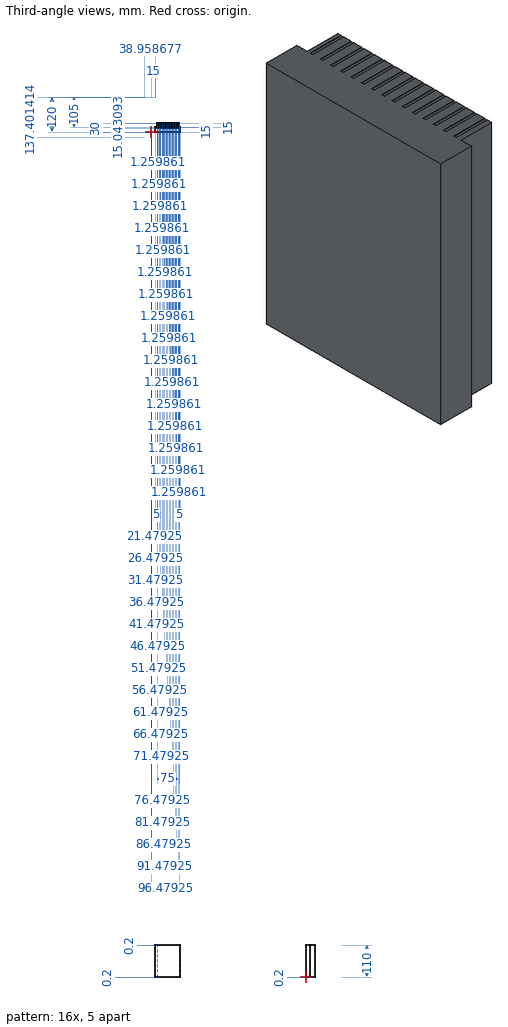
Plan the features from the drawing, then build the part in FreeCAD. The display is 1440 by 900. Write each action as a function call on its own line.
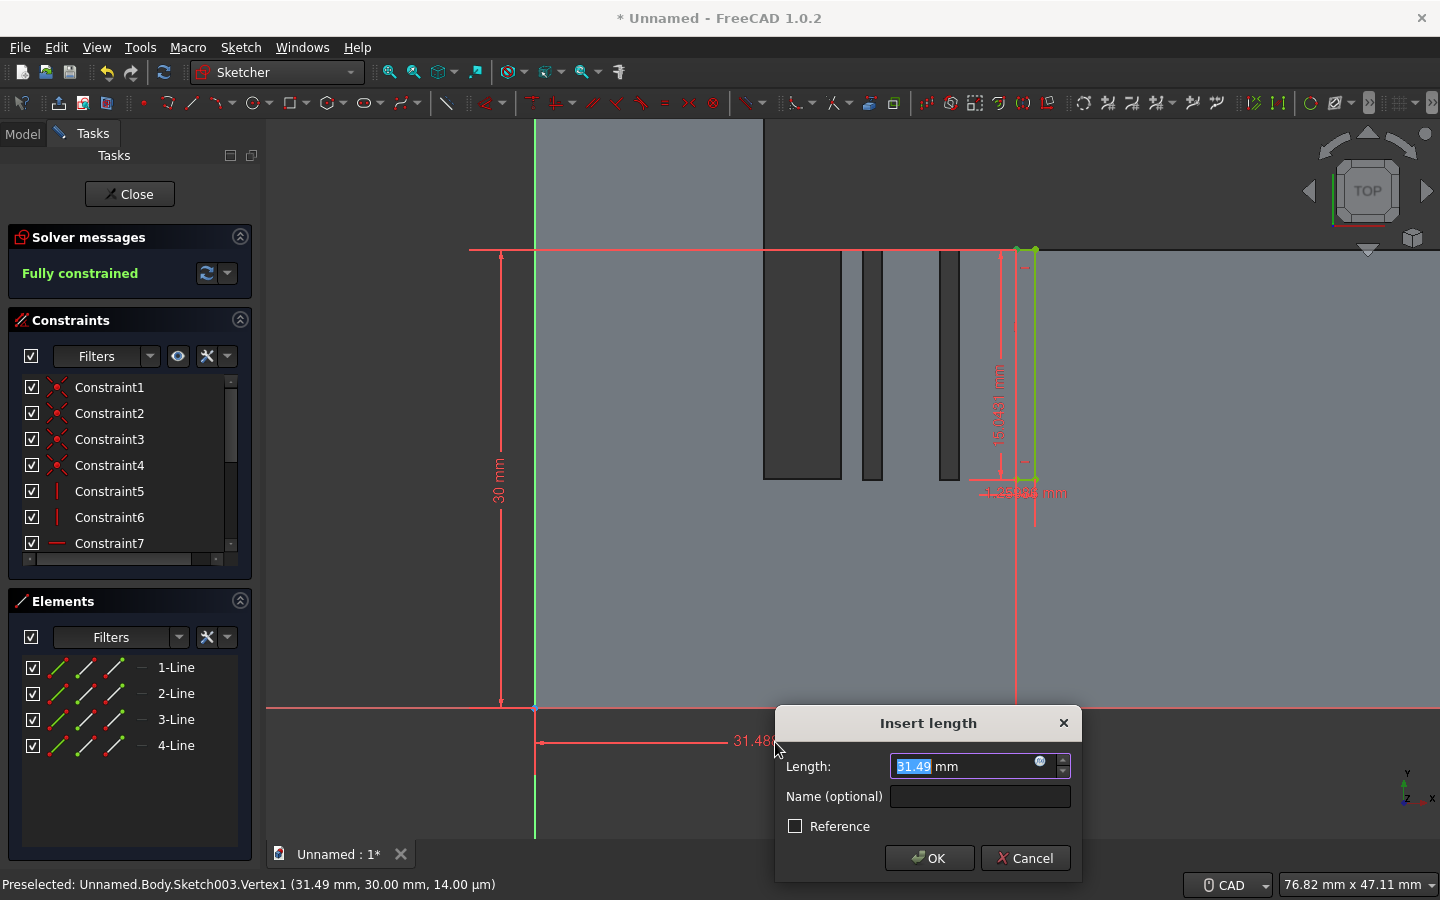
text(31.47925)
key(Return)
key(Escape)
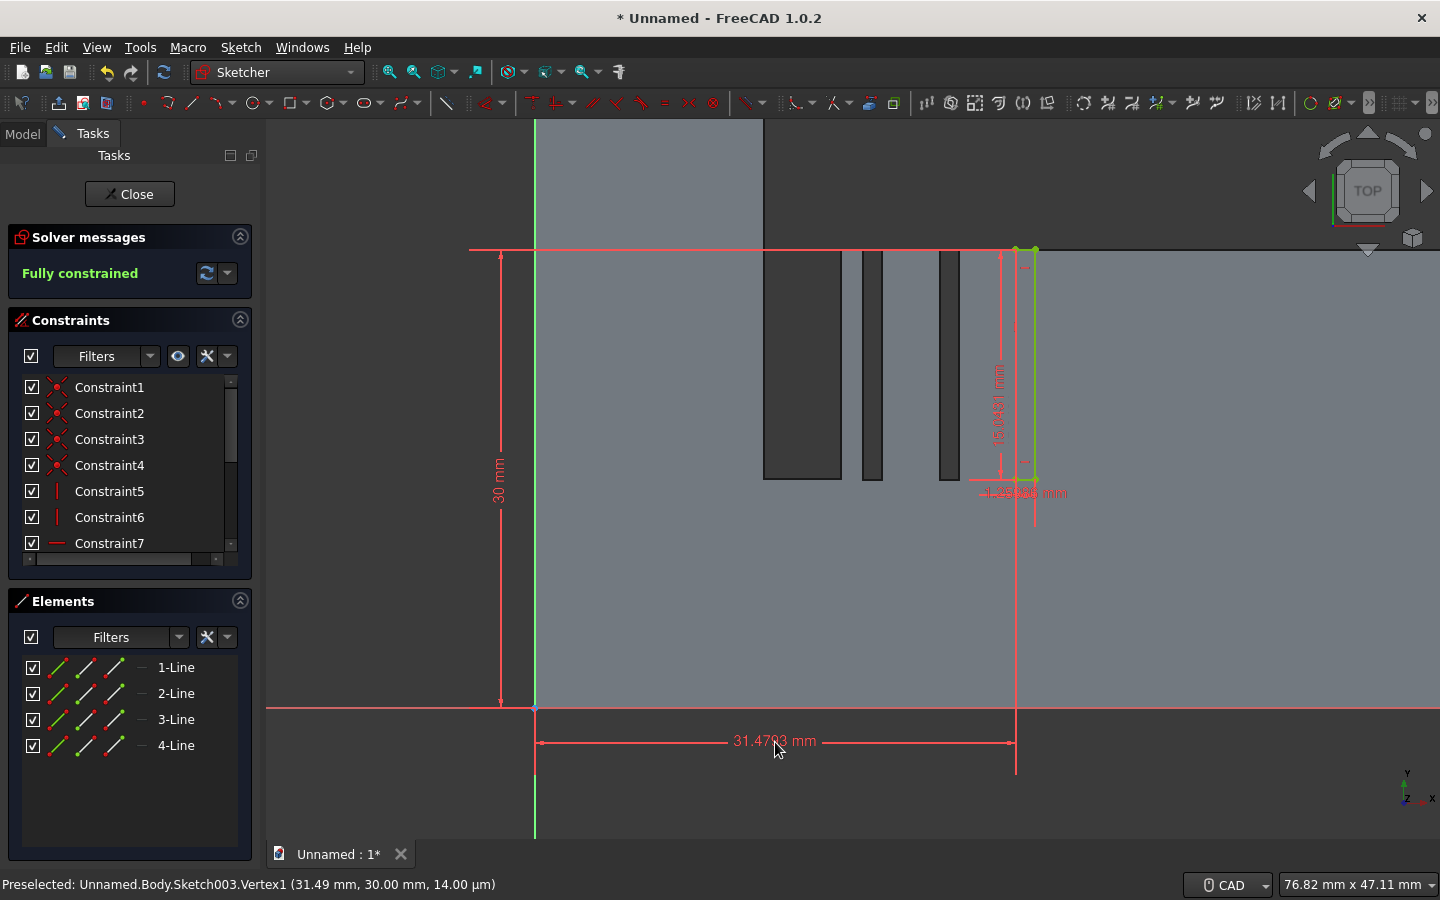
click(130, 194)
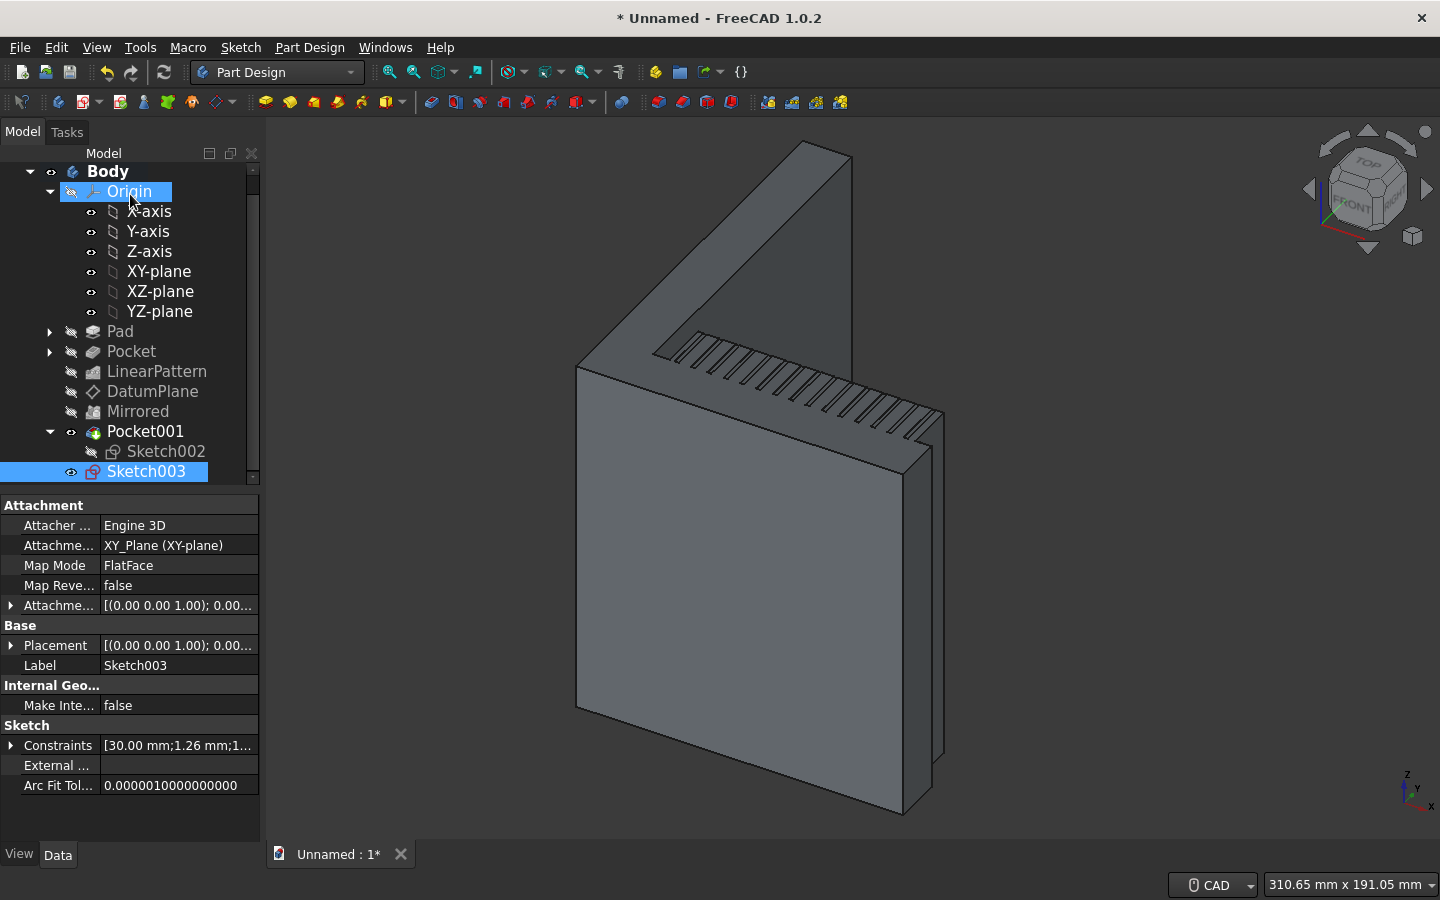
click(432, 102)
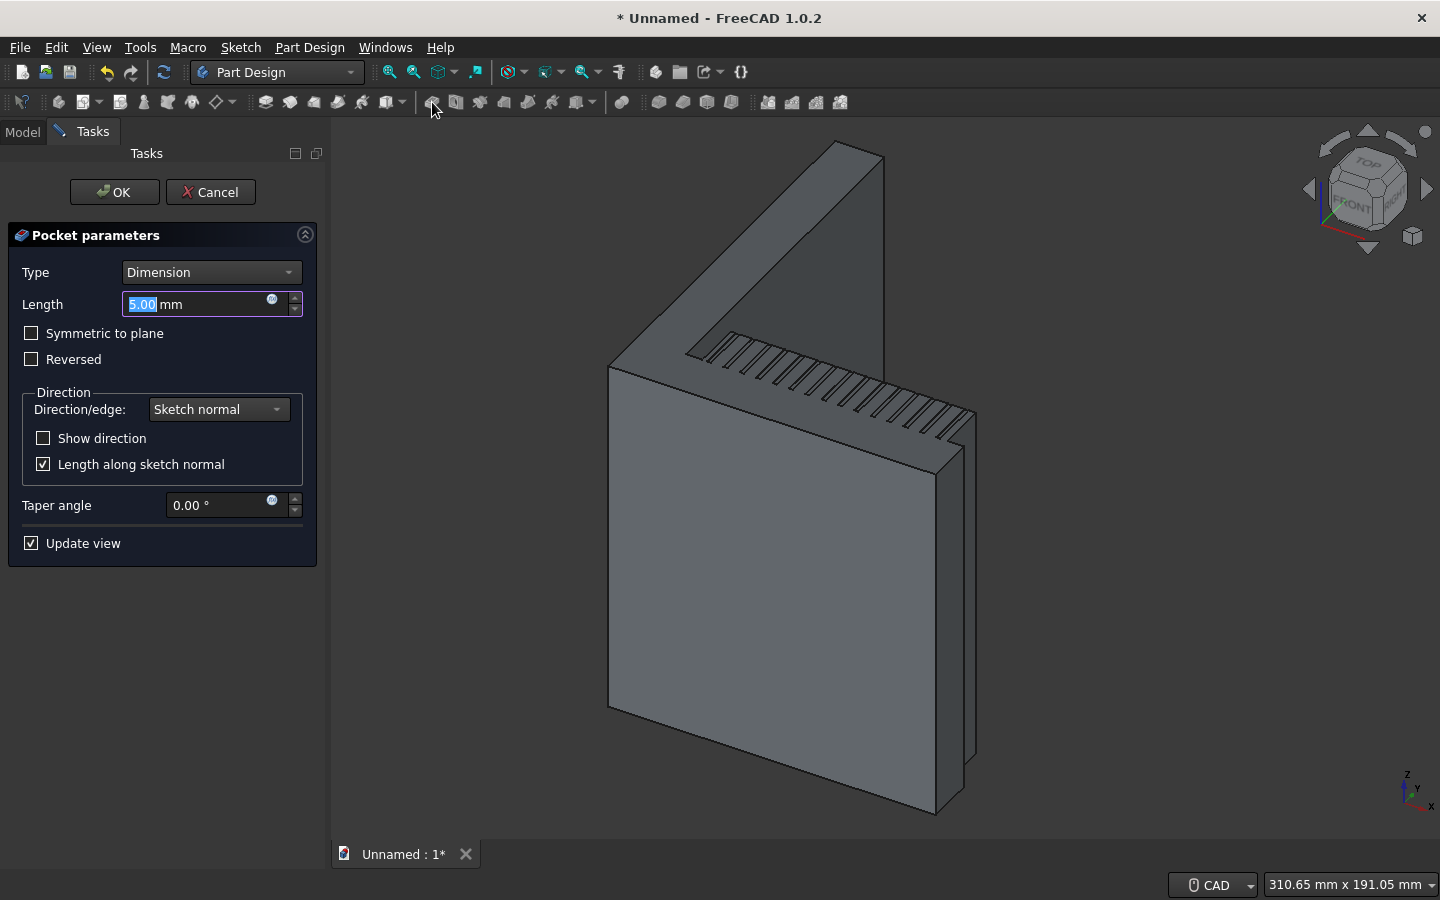
text(0.2)
key(Tab)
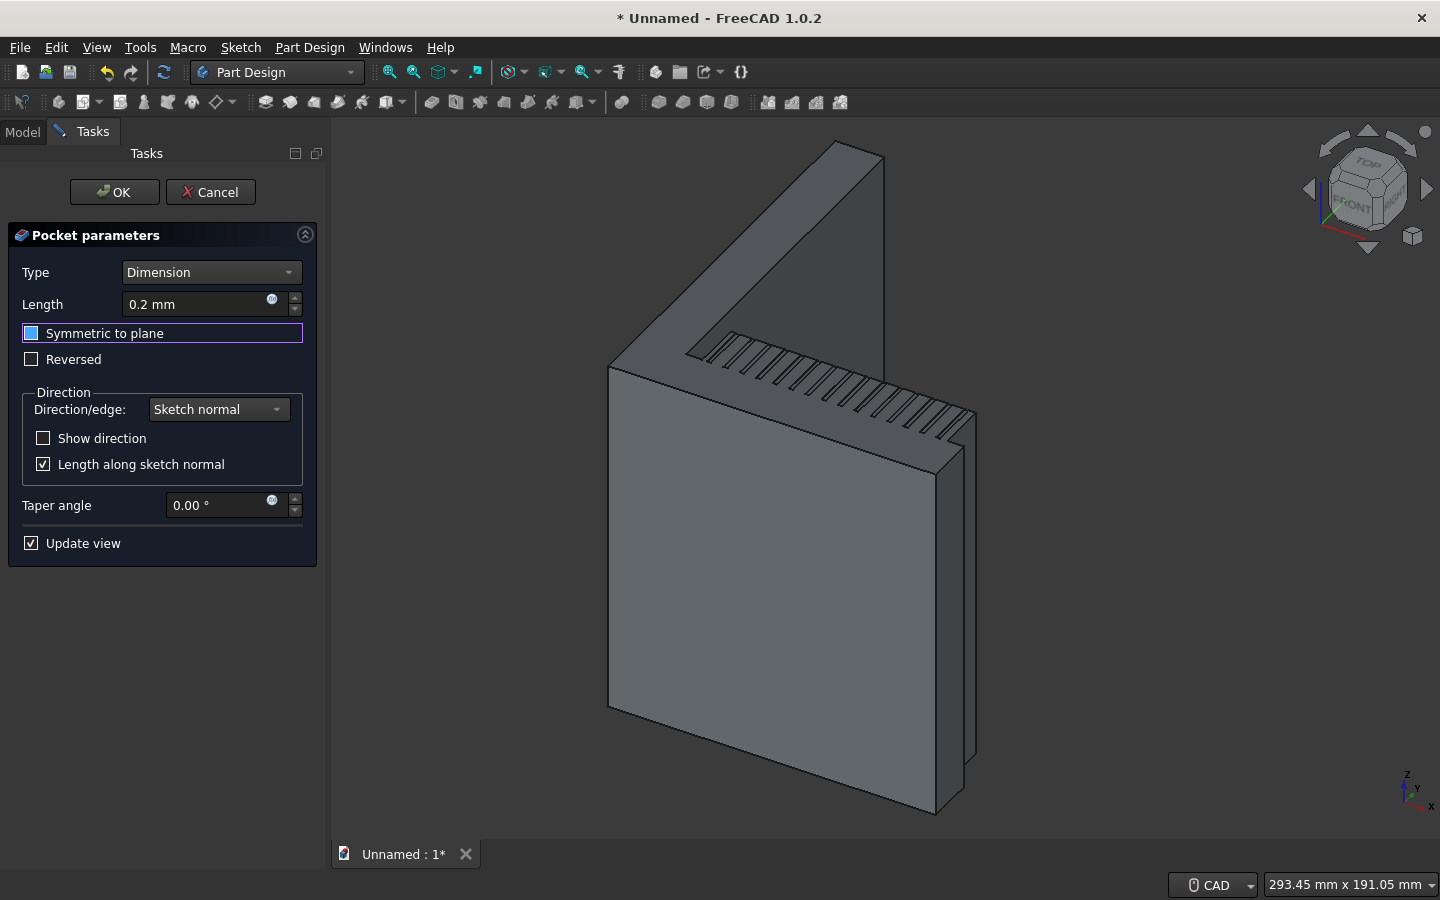
click(30, 359)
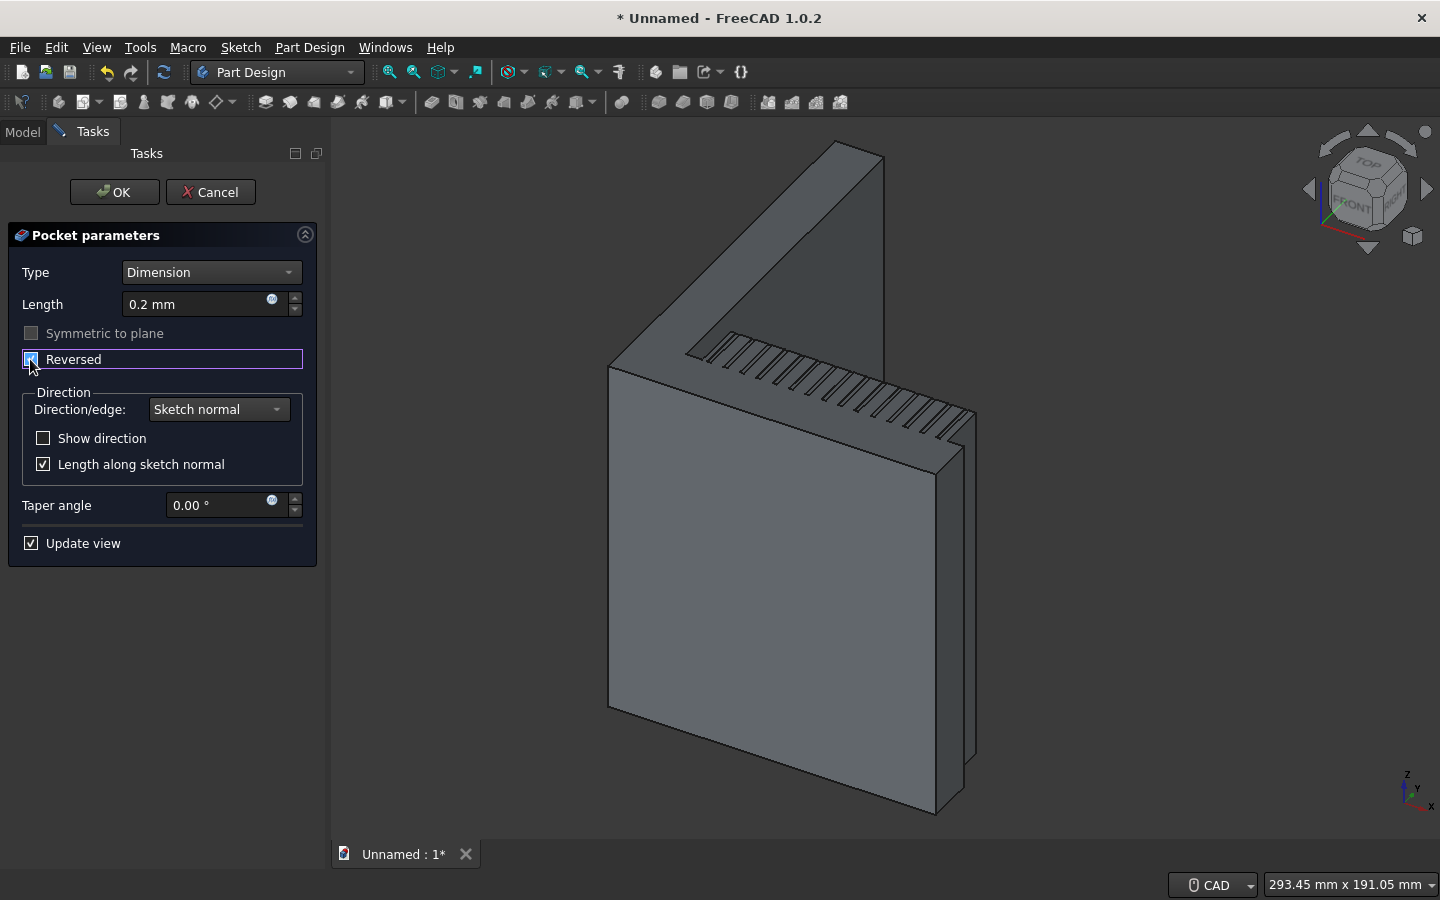
click(115, 192)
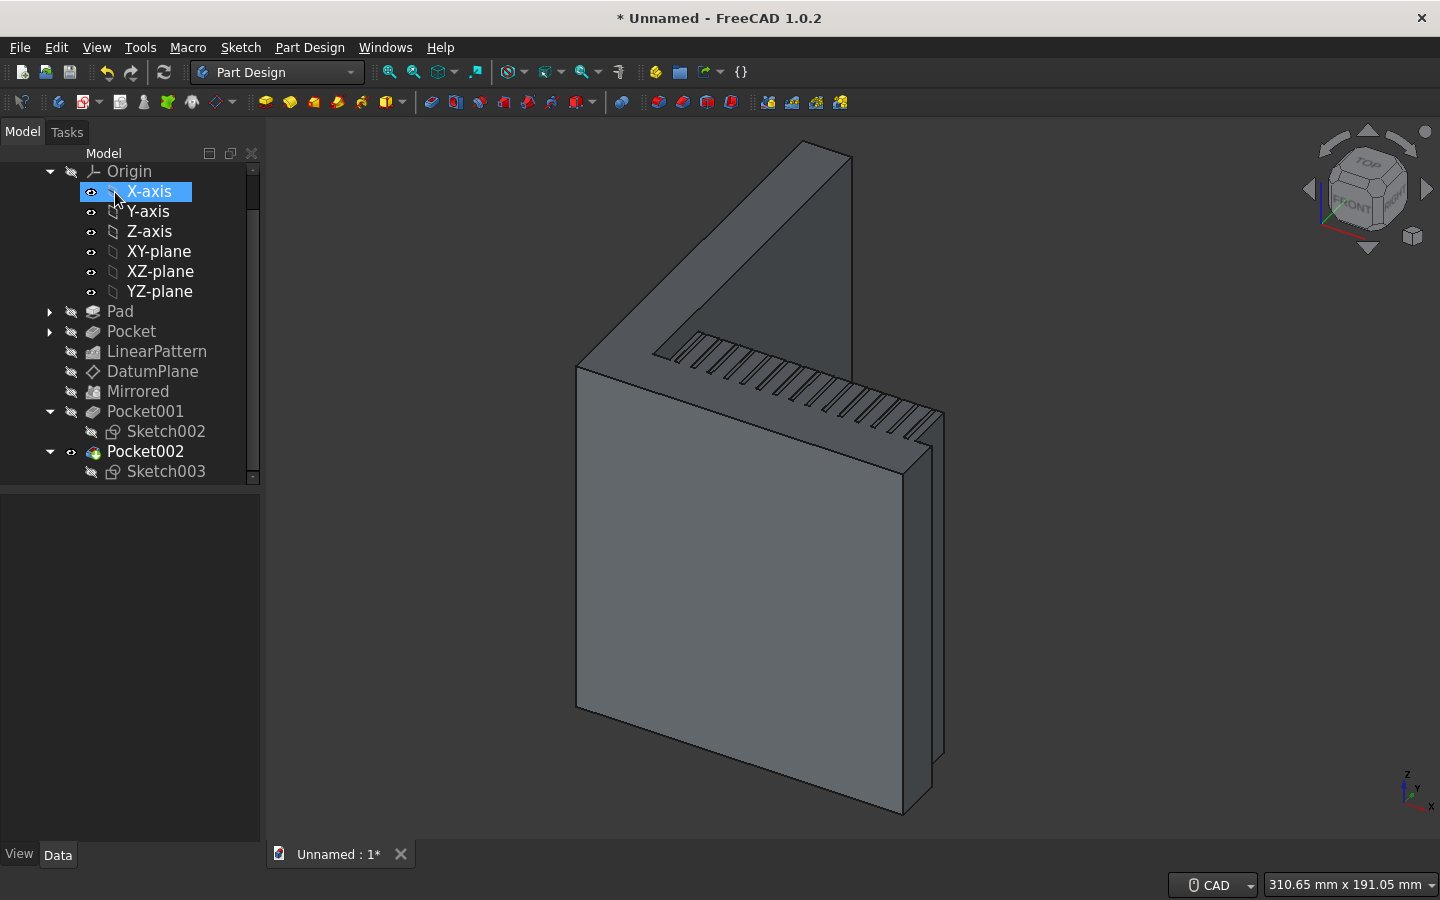
key(5)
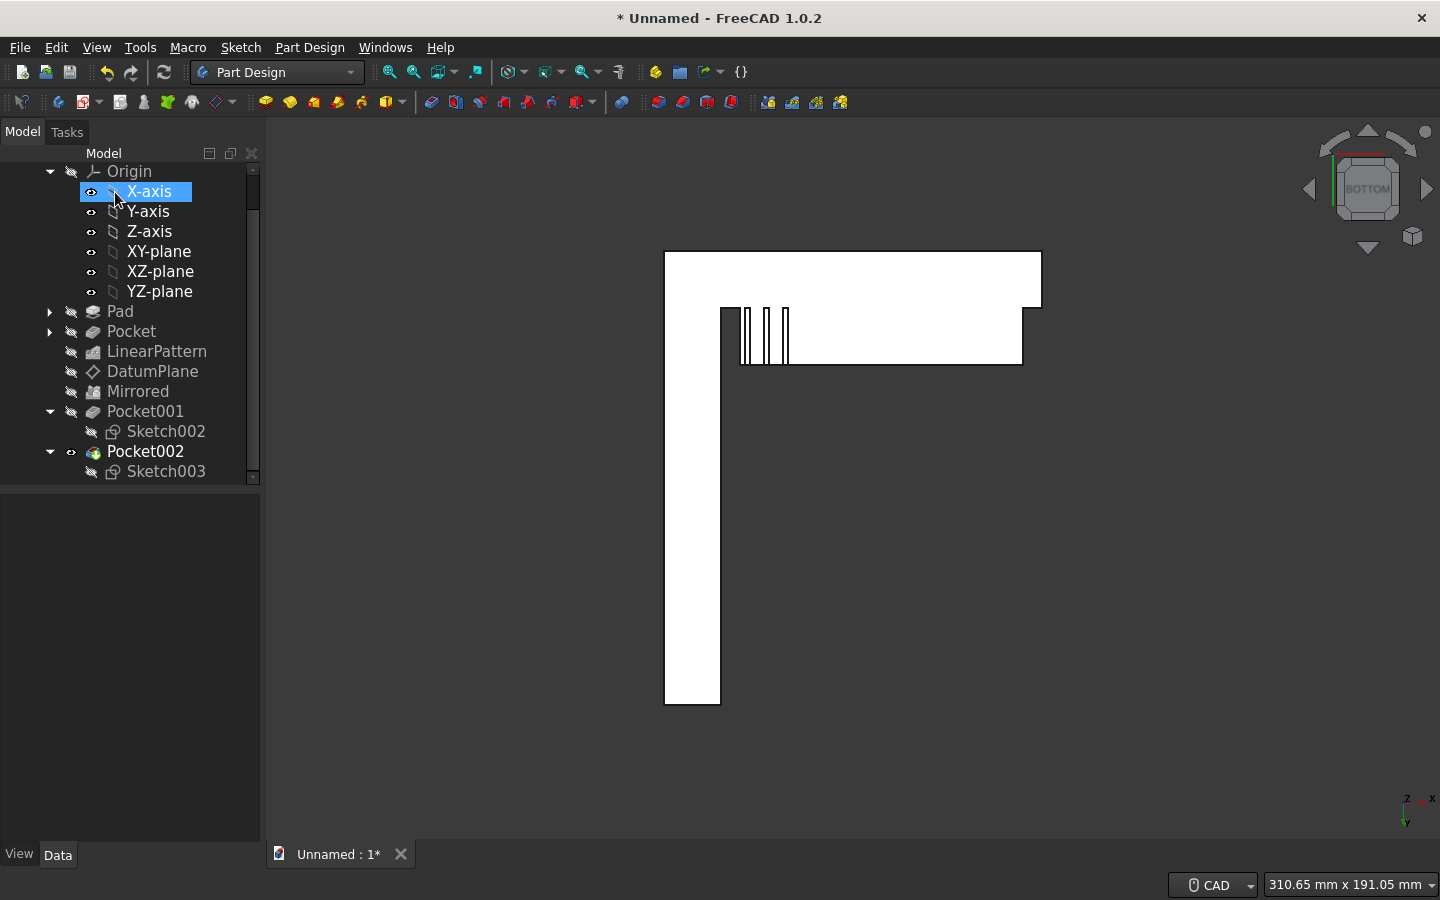
click(961, 283)